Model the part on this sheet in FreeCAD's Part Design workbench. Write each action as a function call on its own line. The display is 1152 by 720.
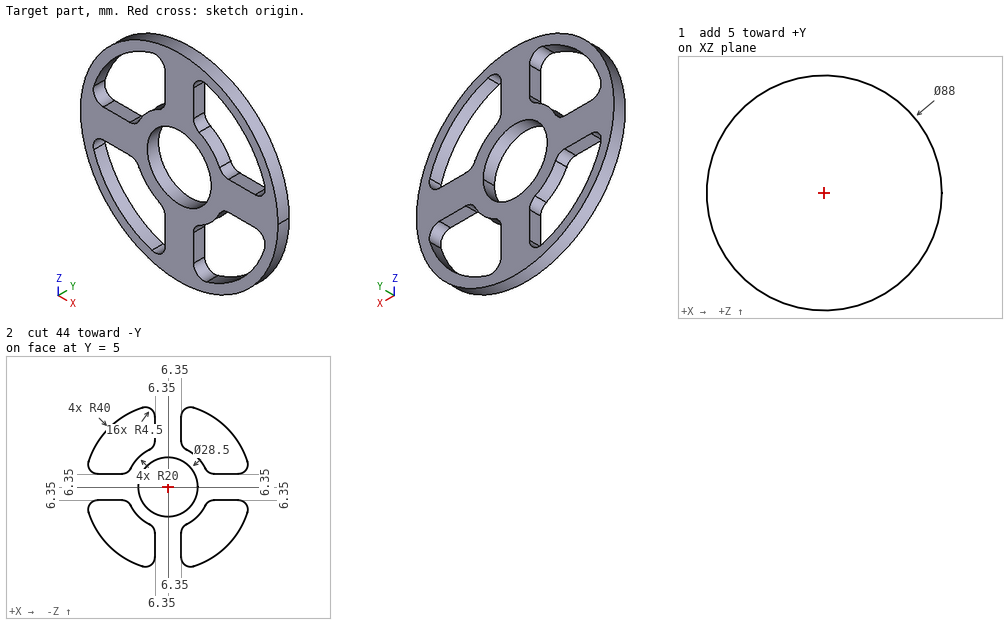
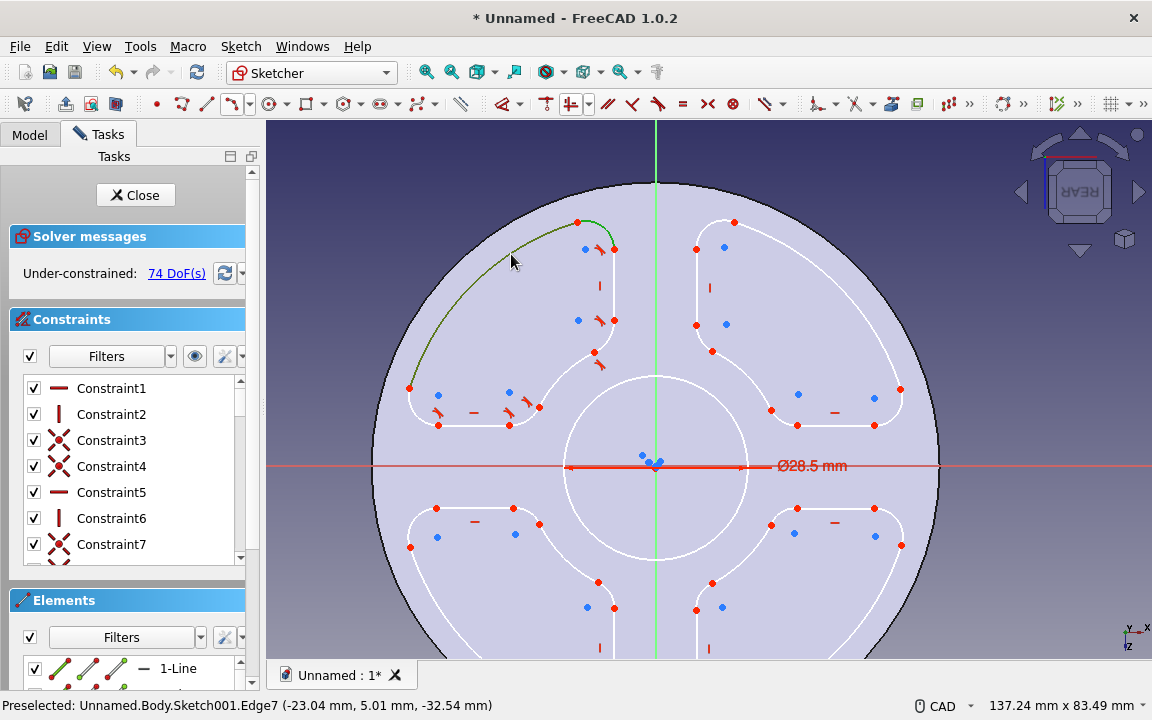
key(t)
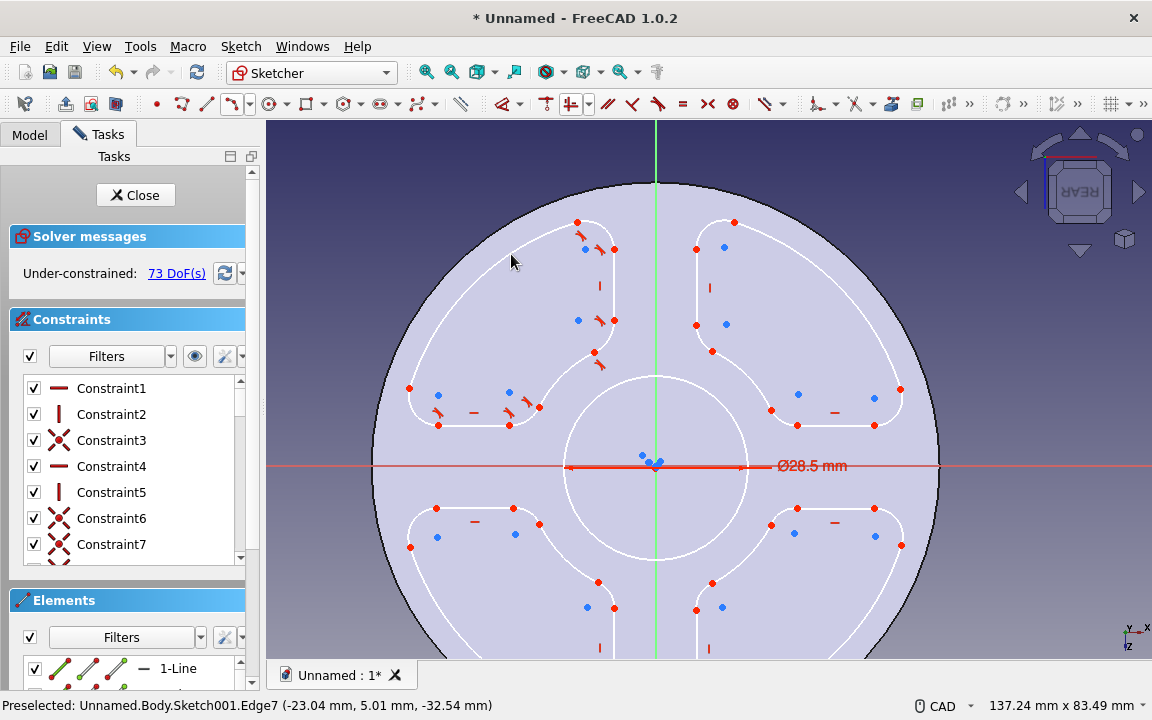
click(511, 254)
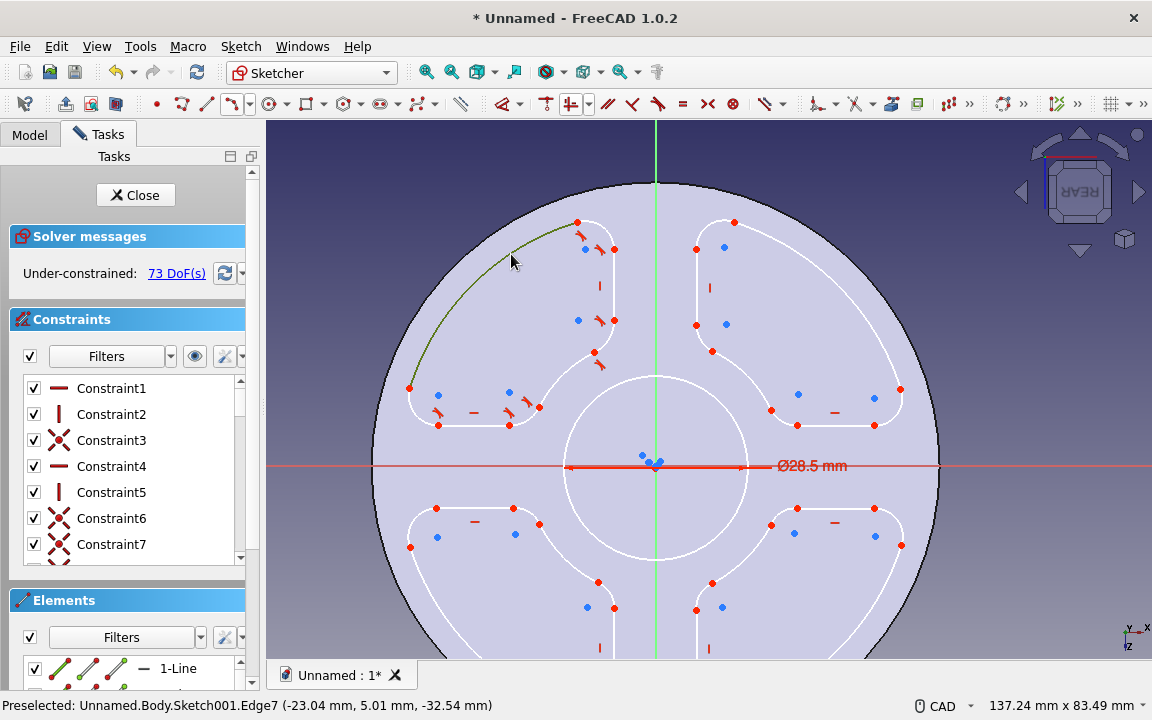
click(410, 404)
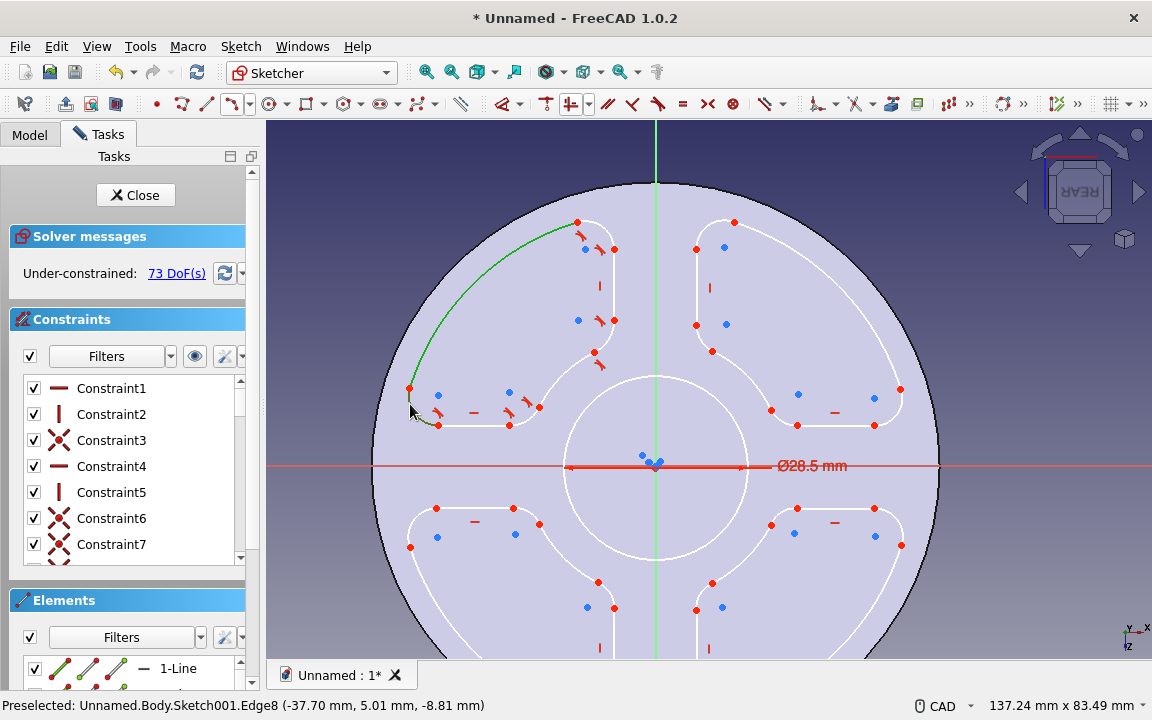
click(658, 104)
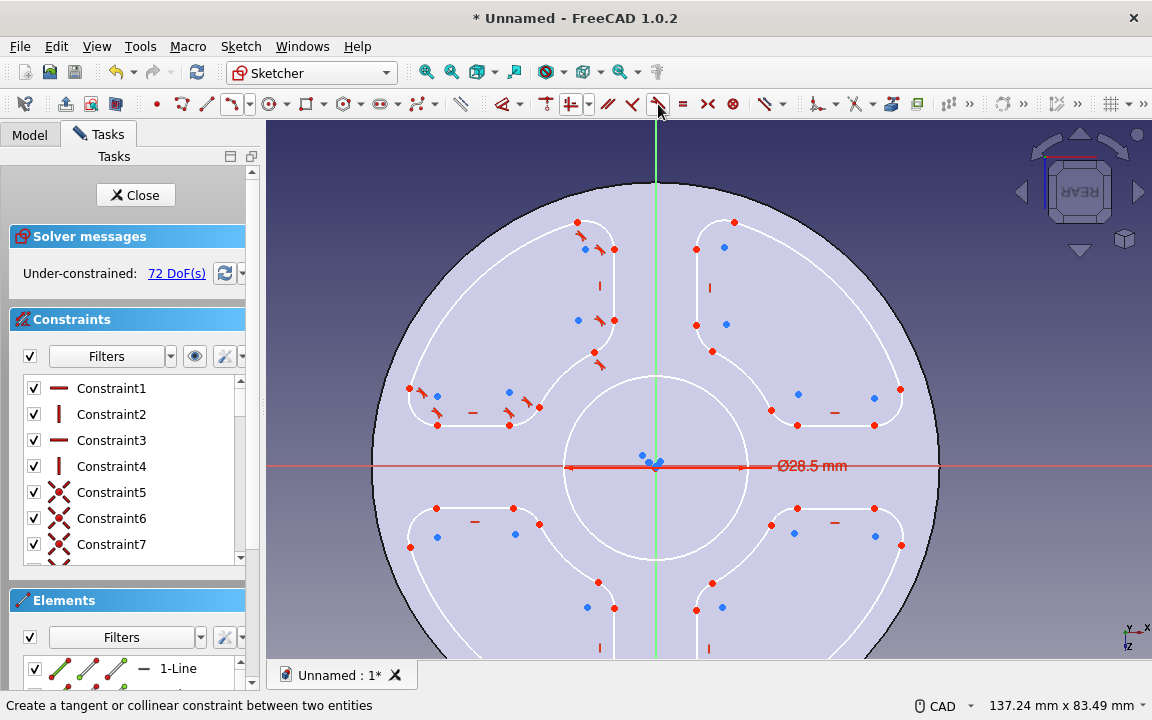
click(820, 426)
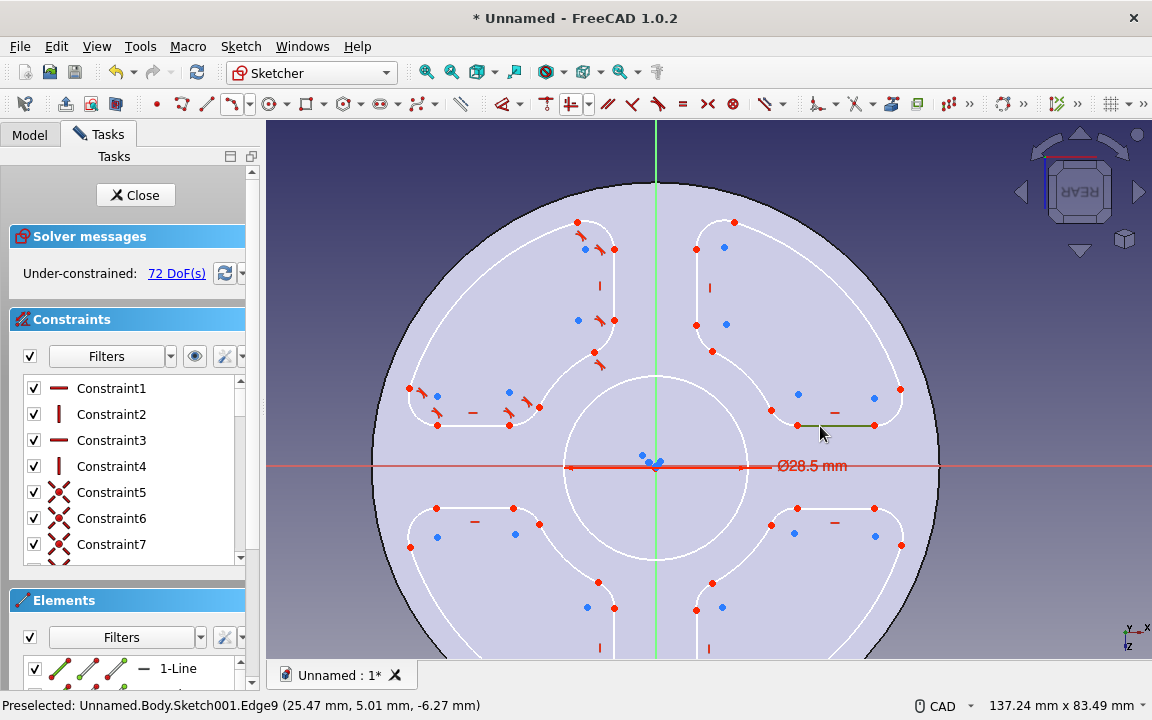
click(889, 422)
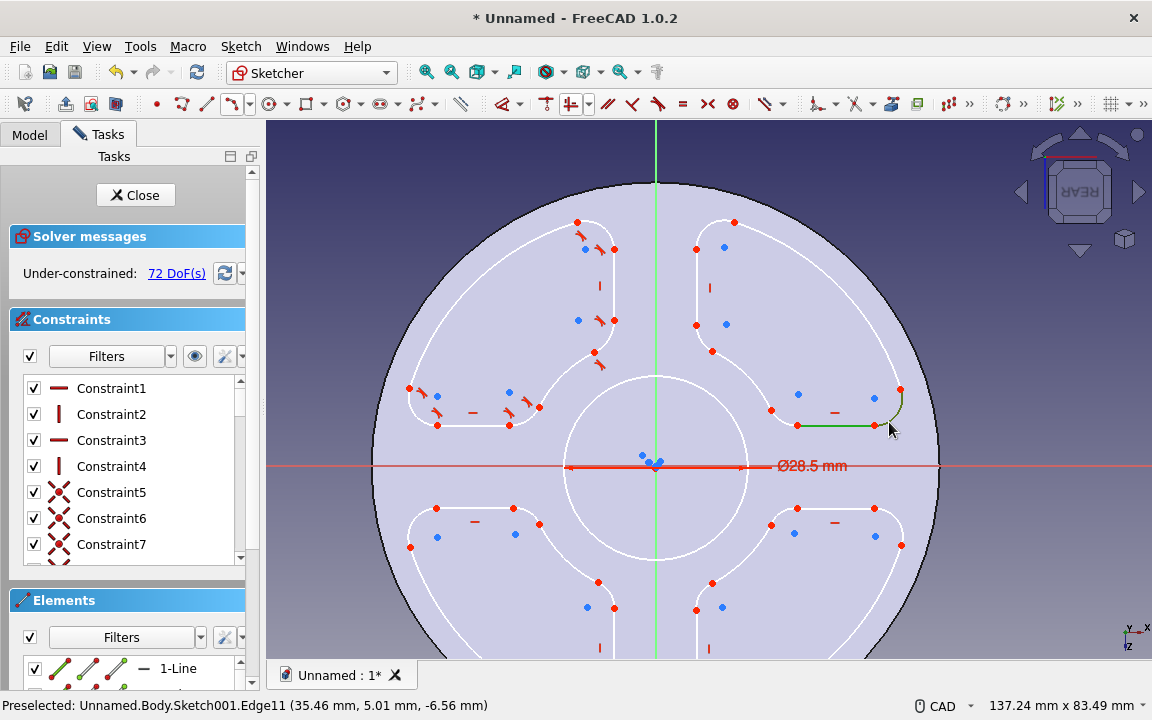
key(t)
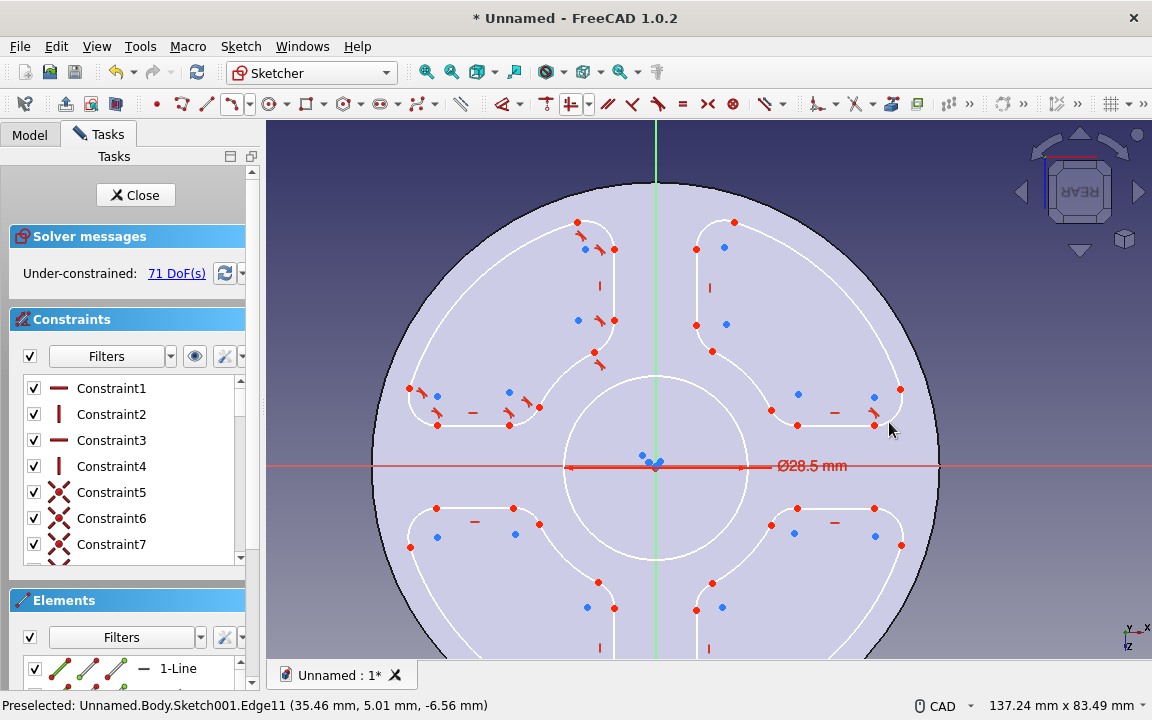
click(820, 426)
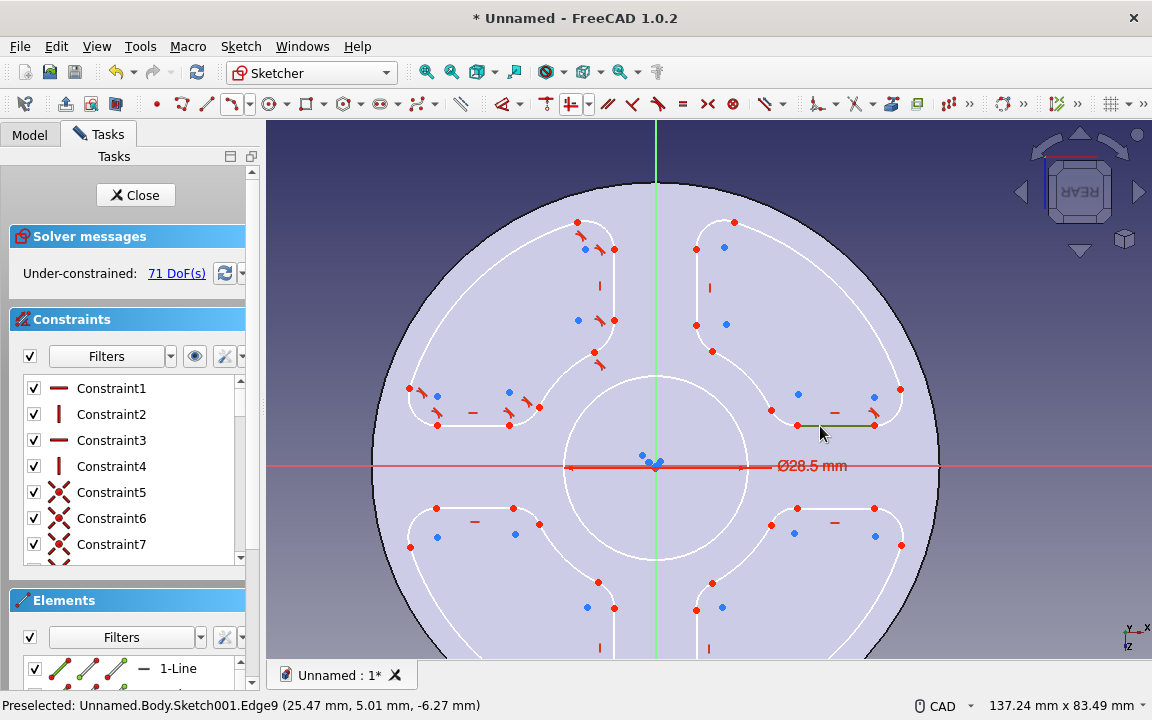
scroll(777, 418, up, 2)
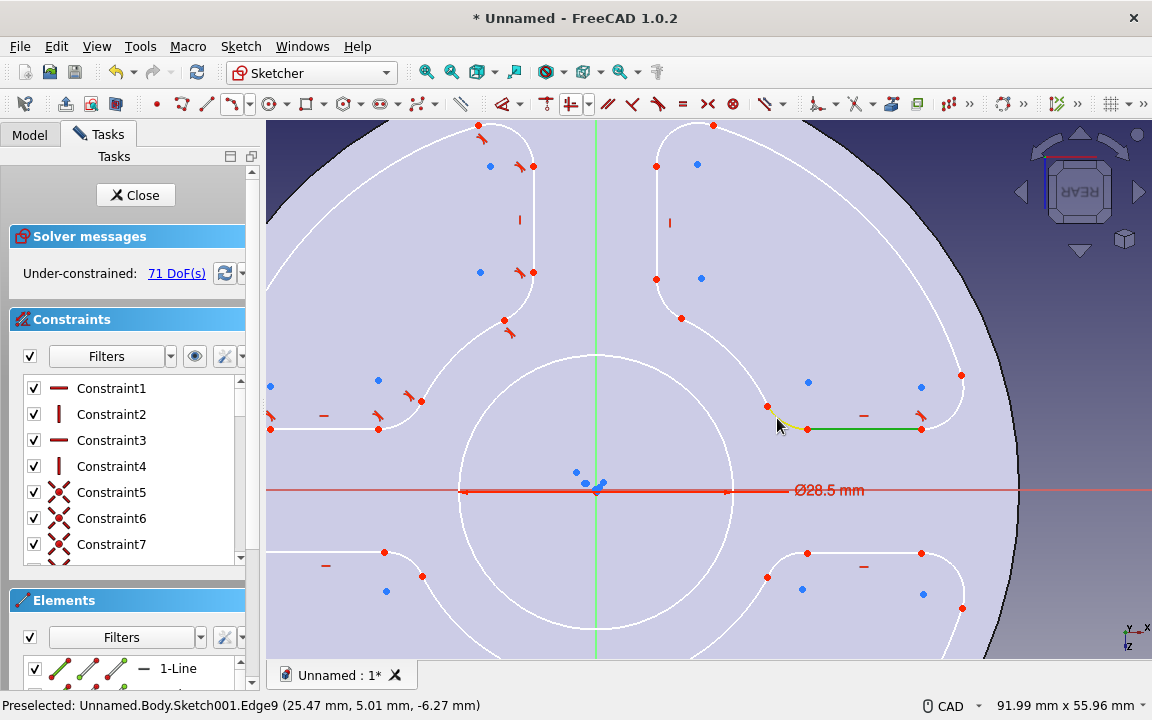
click(777, 417)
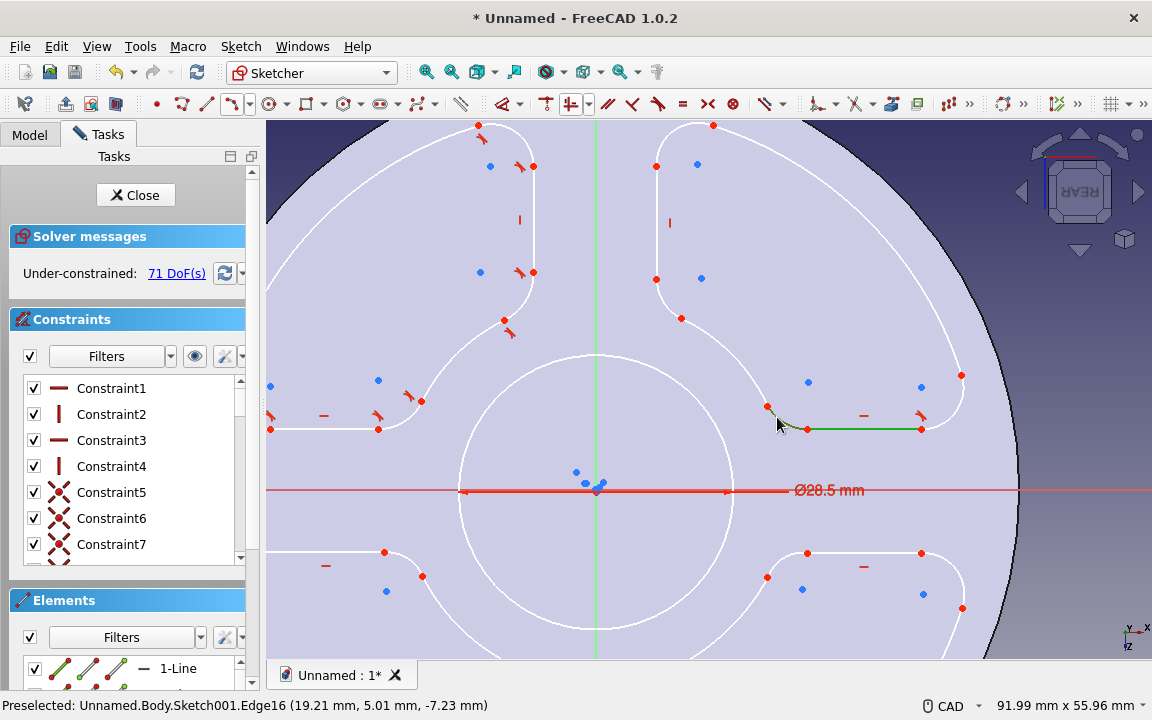
click(658, 104)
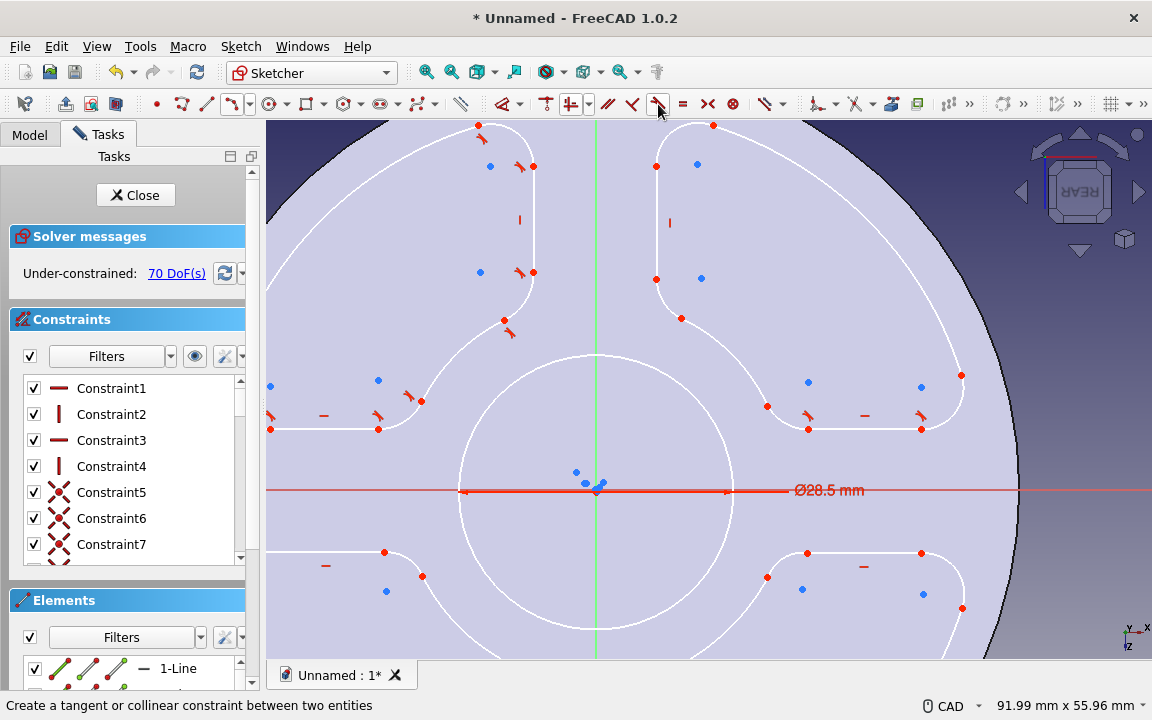
click(657, 200)